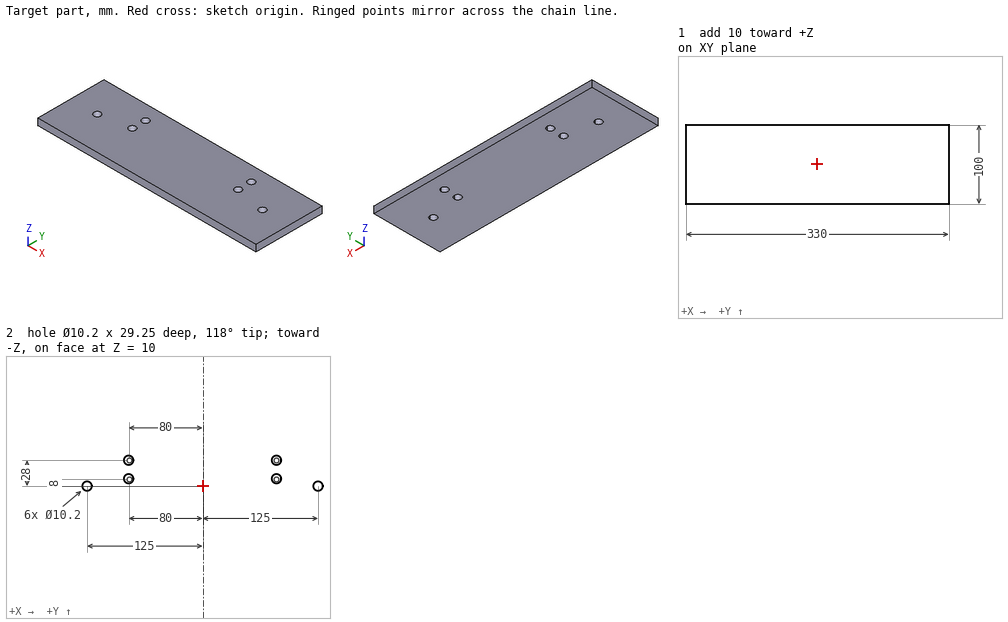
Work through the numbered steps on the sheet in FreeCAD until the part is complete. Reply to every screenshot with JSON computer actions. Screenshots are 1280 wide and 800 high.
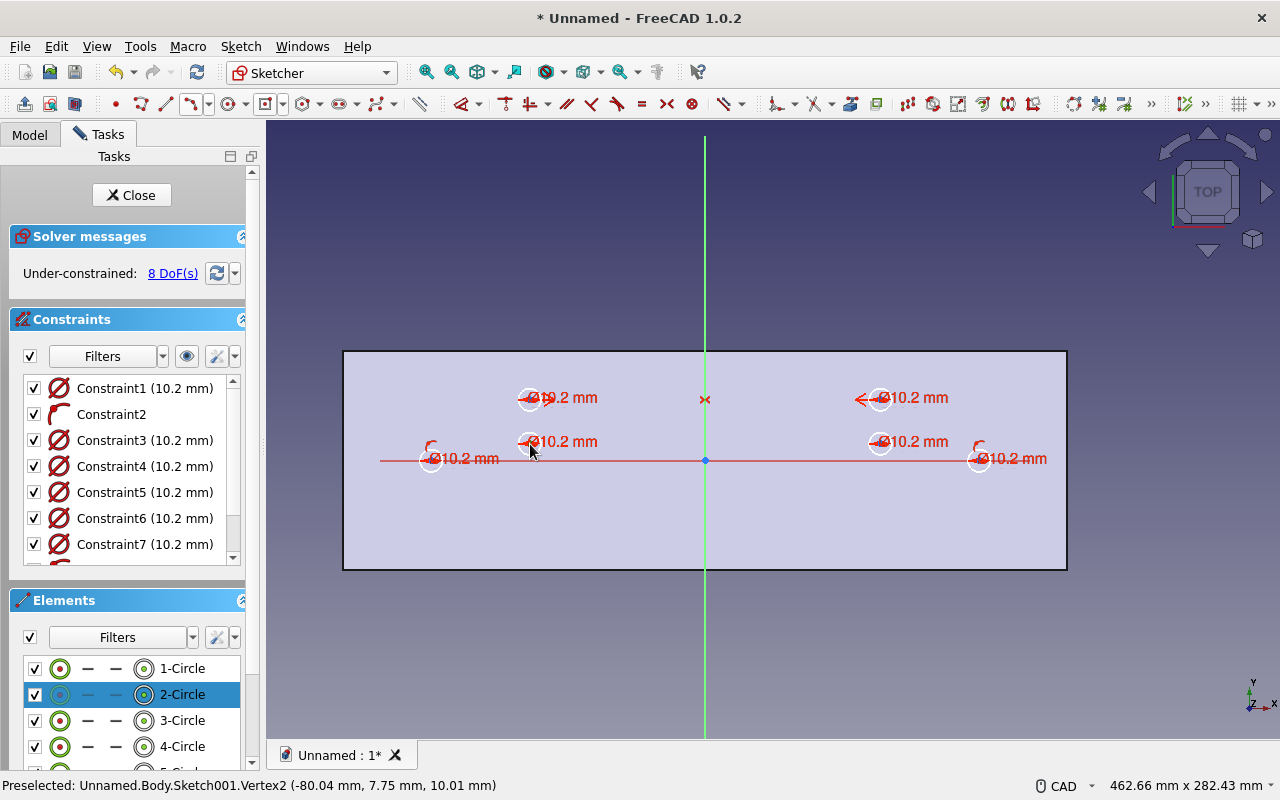
{"action": "left_click", "coordinate": [880, 444]}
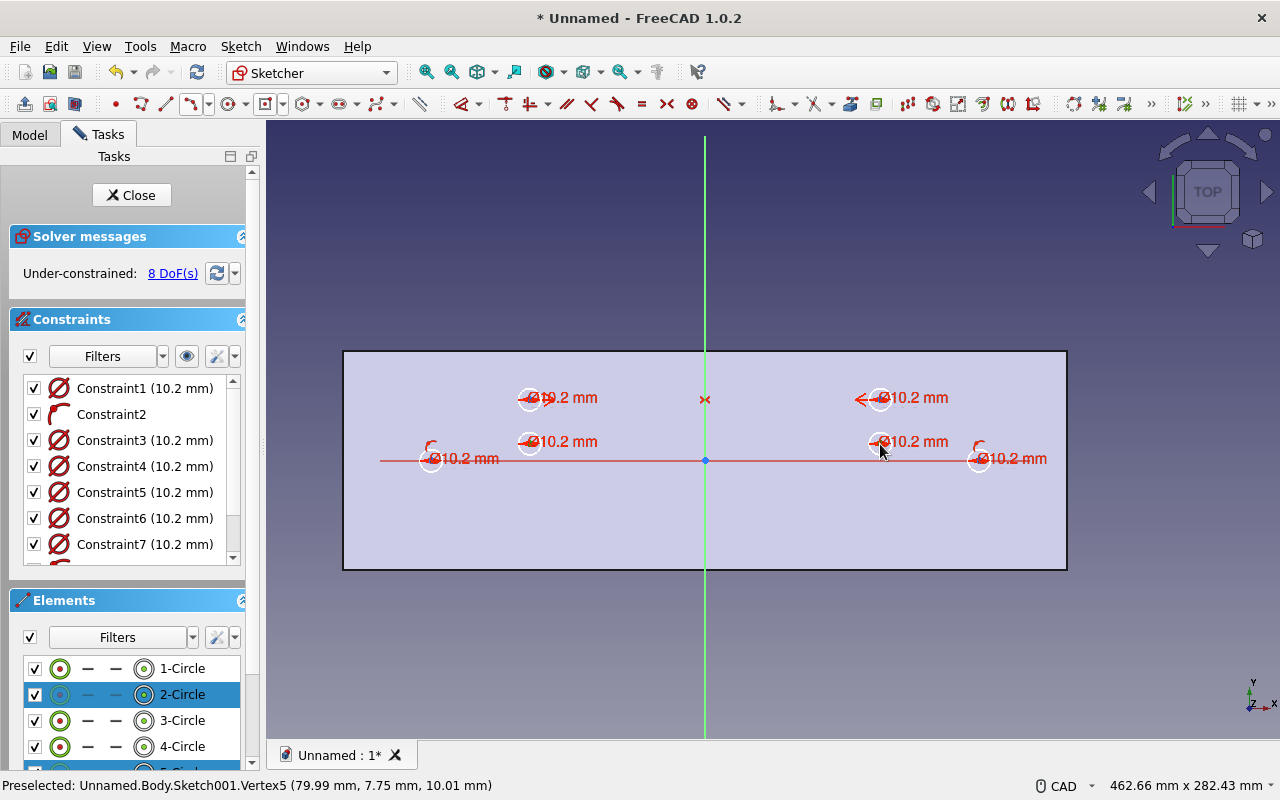
{"action": "left_click", "coordinate": [705, 671]}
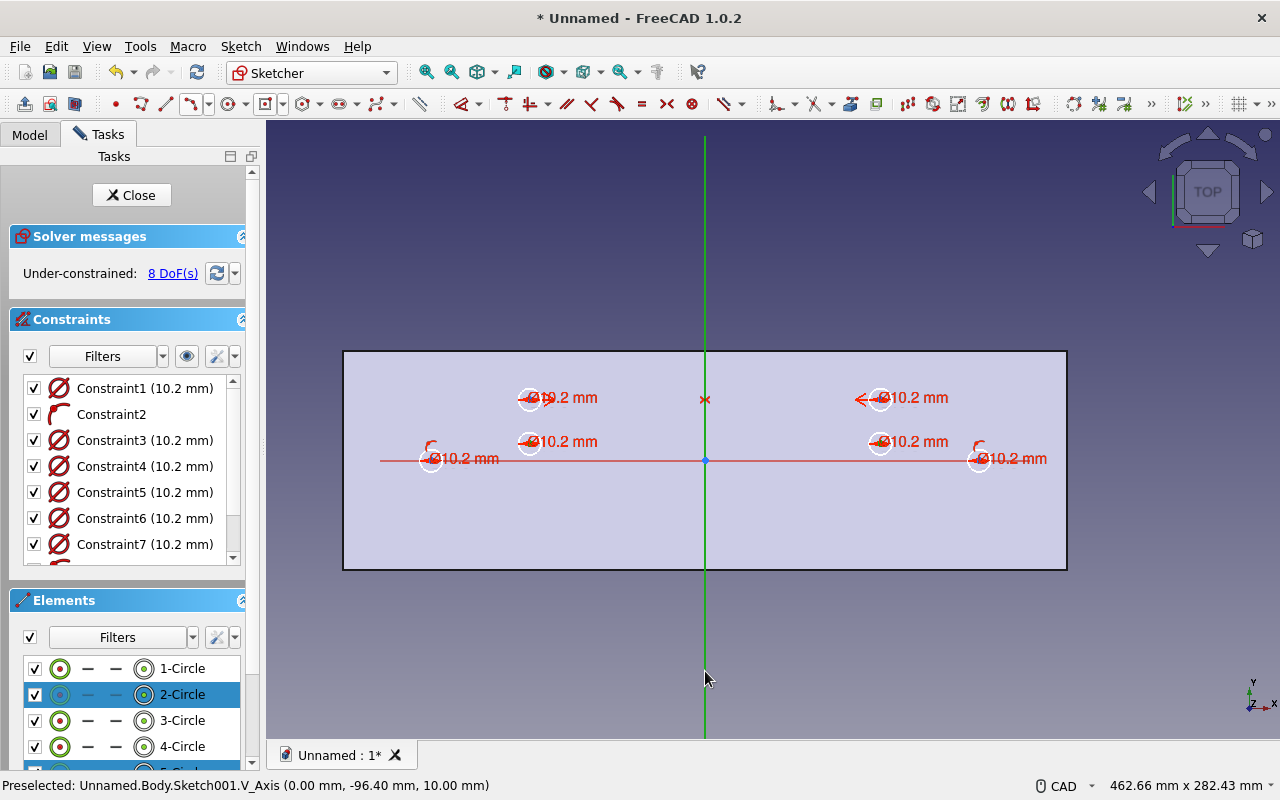
{"action": "left_click", "coordinate": [667, 104]}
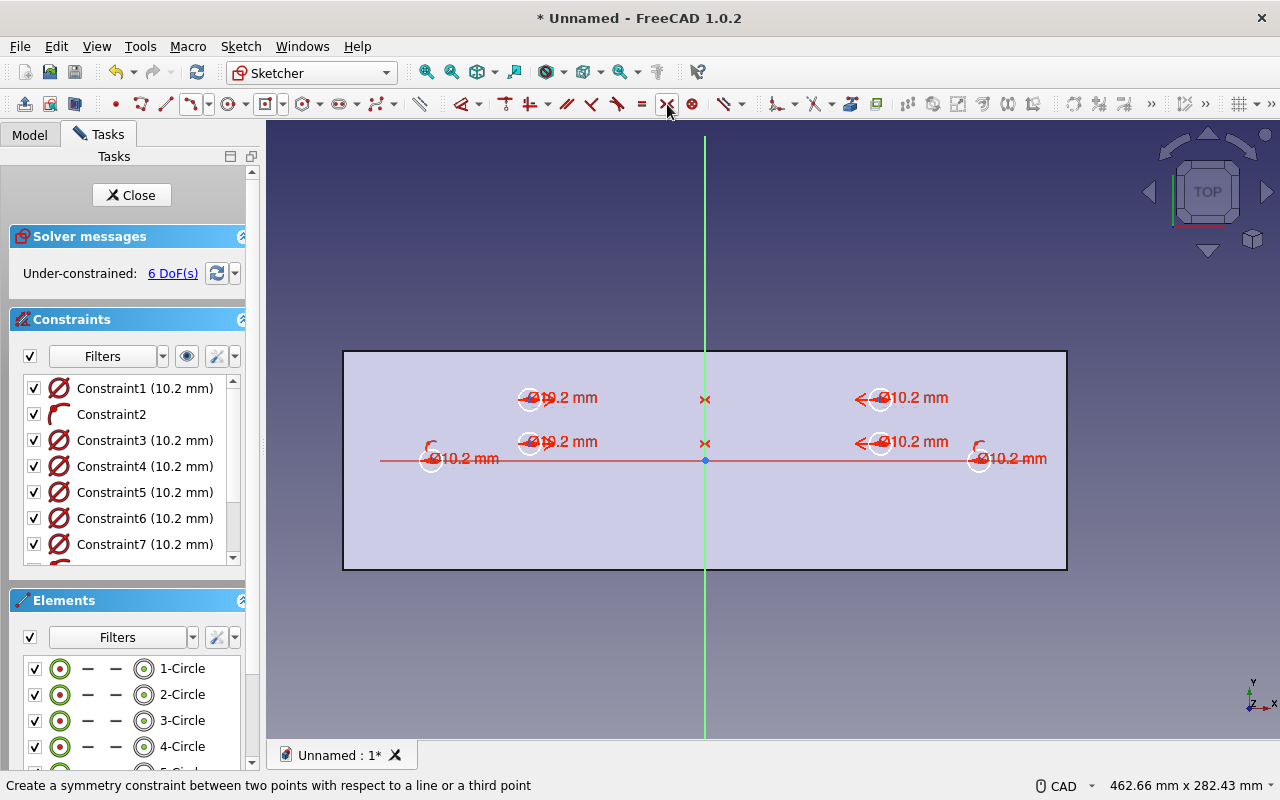
{"action": "scroll", "coordinate": [530, 444], "scroll_direction": "up", "scroll_amount": 5}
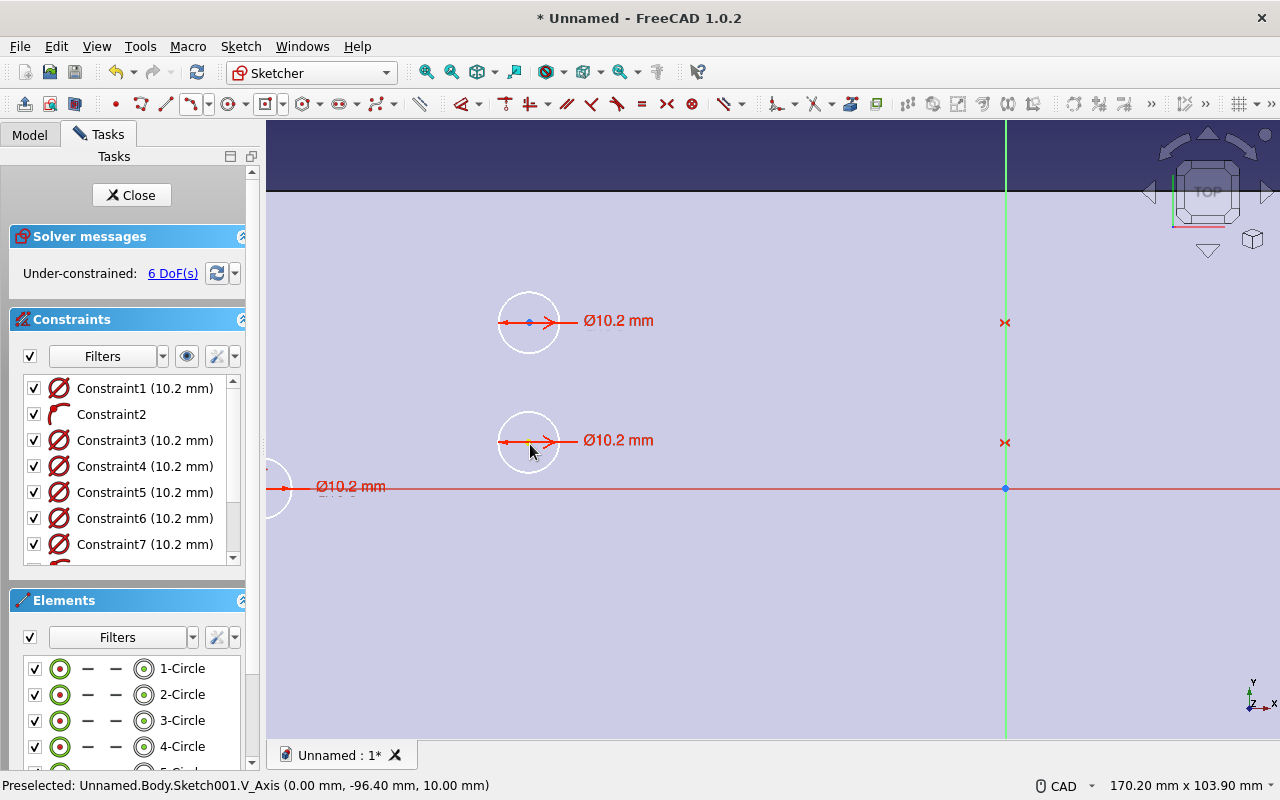
{"action": "left_click", "coordinate": [529, 442]}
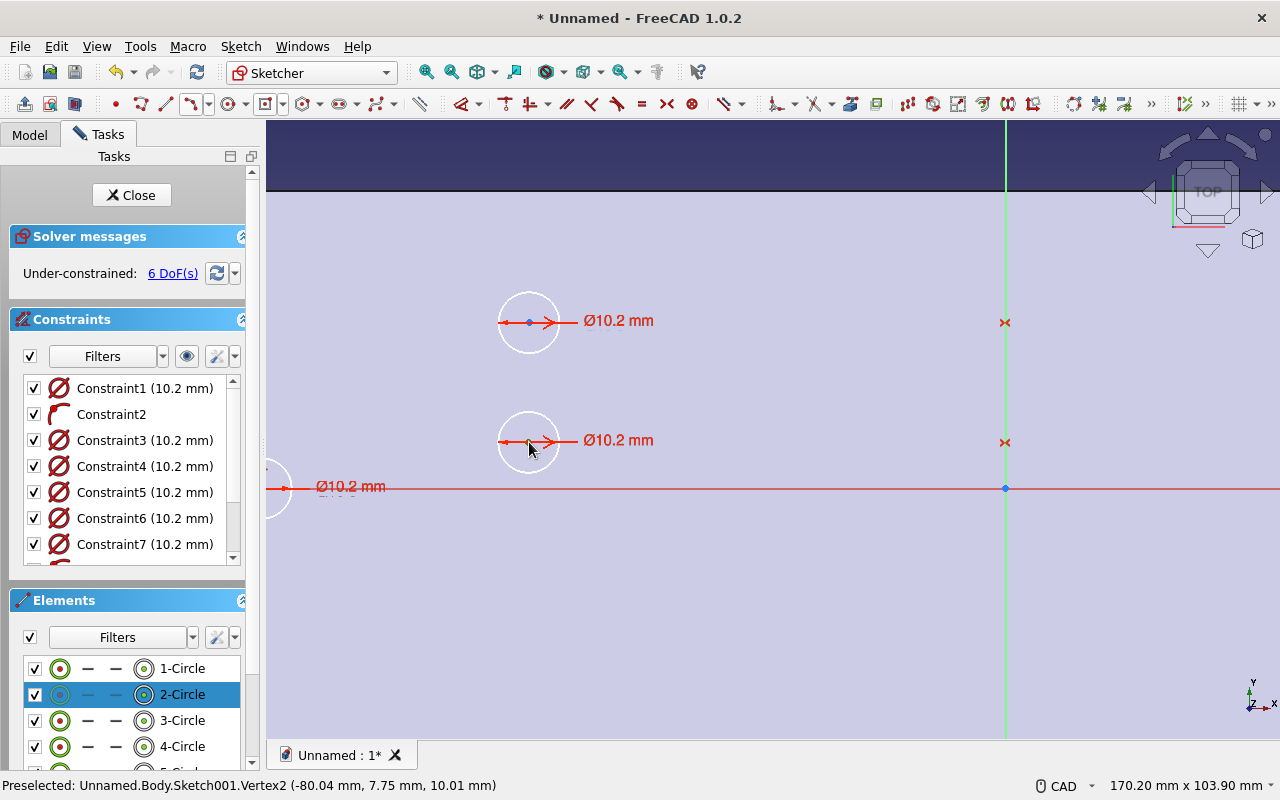
{"action": "key", "text": "i"}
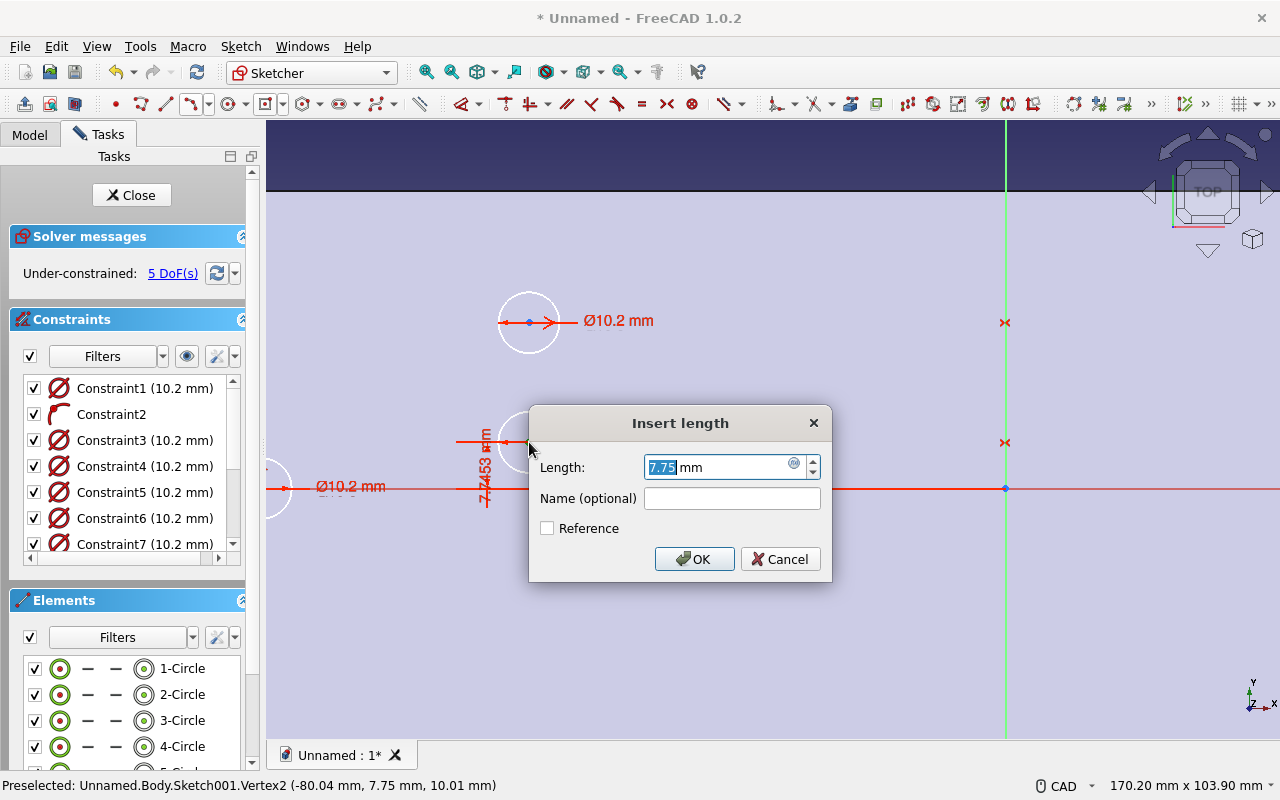
{"action": "type", "text": "8"}
{"action": "key", "text": "Return"}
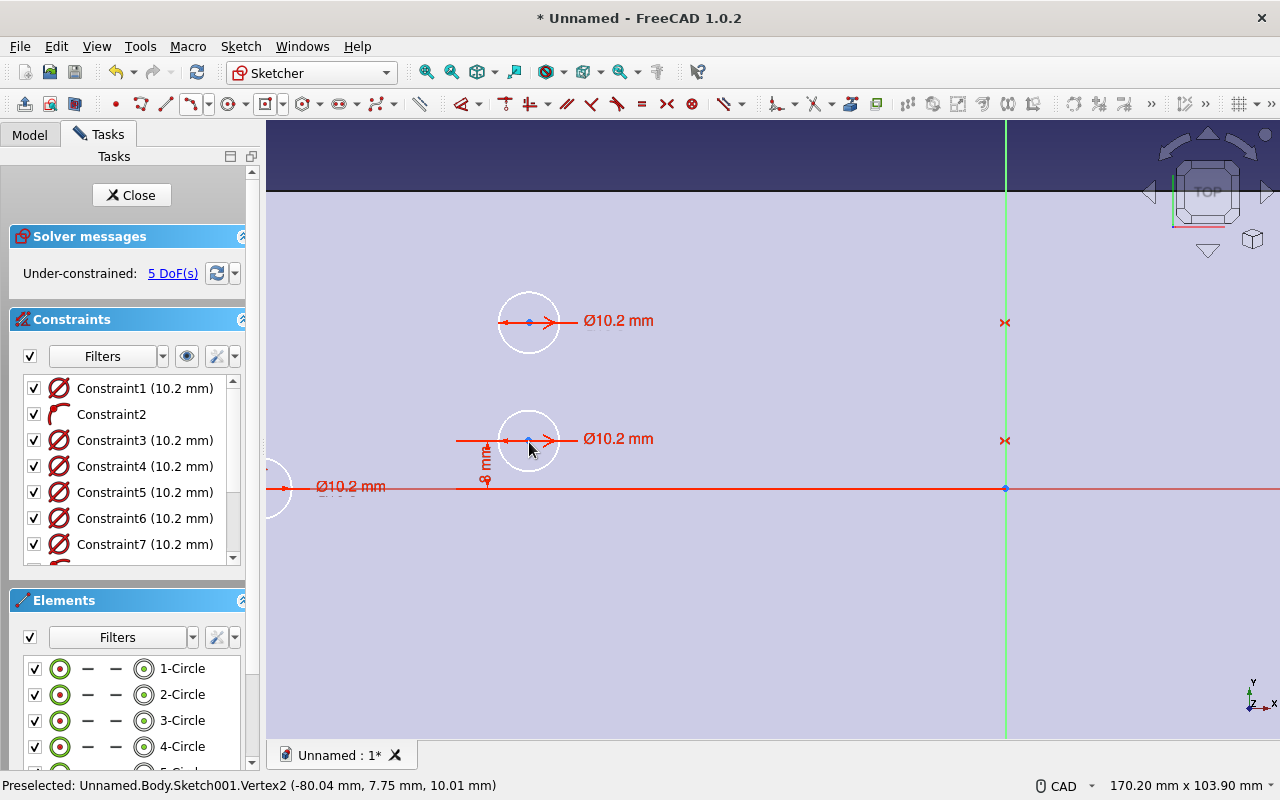
{"action": "left_click", "coordinate": [529, 441]}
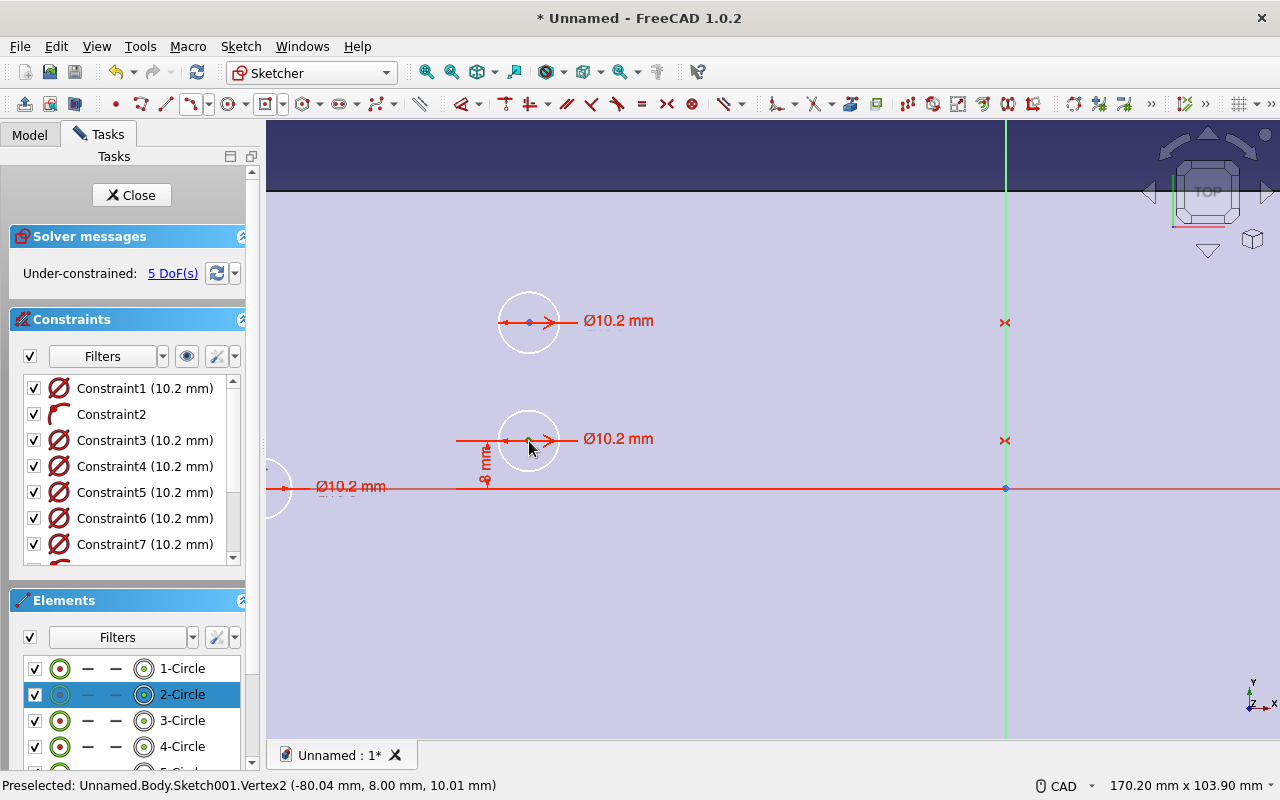
{"action": "left_click", "coordinate": [478, 104]}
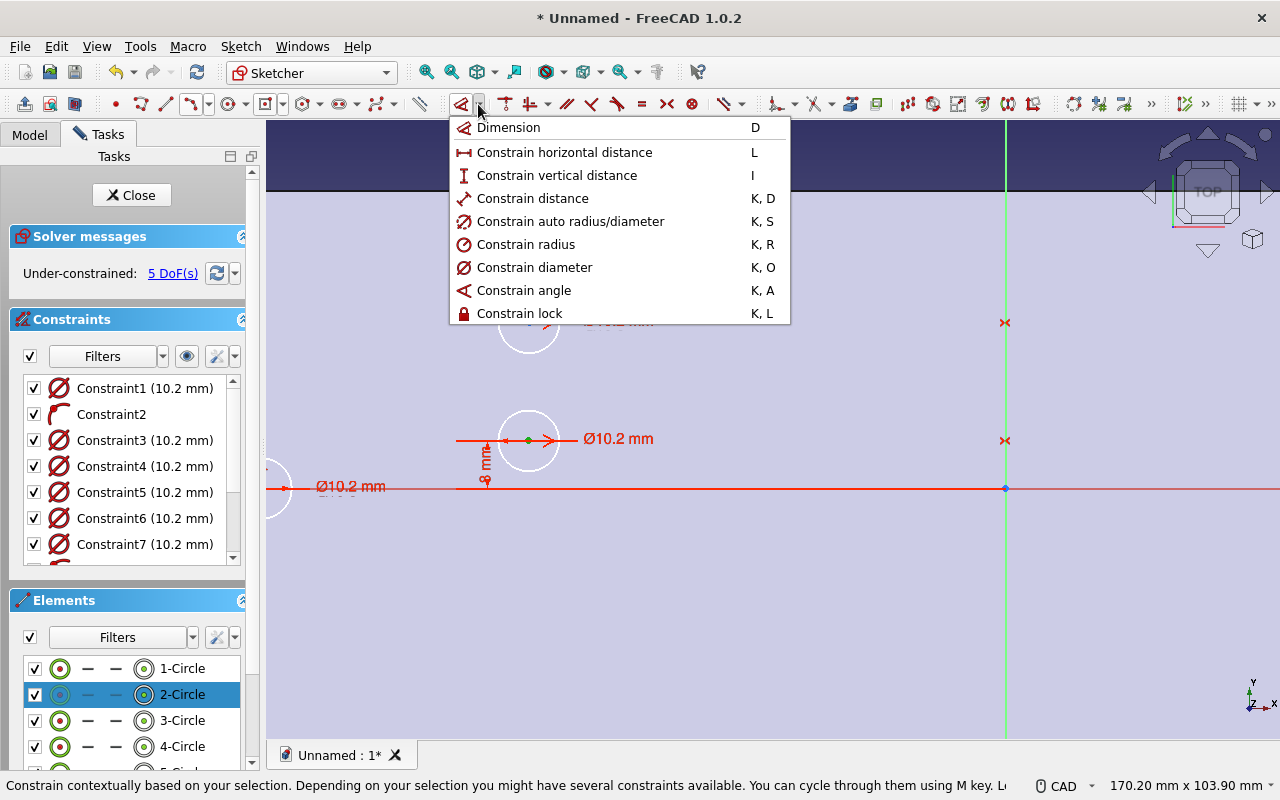
{"action": "left_click", "coordinate": [620, 152]}